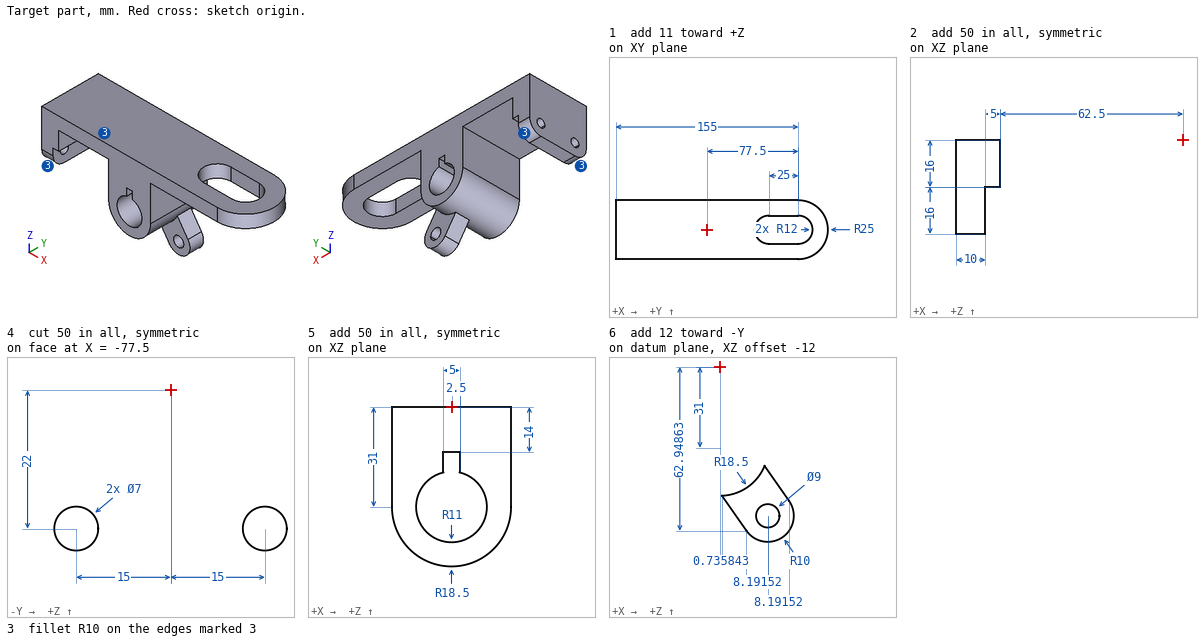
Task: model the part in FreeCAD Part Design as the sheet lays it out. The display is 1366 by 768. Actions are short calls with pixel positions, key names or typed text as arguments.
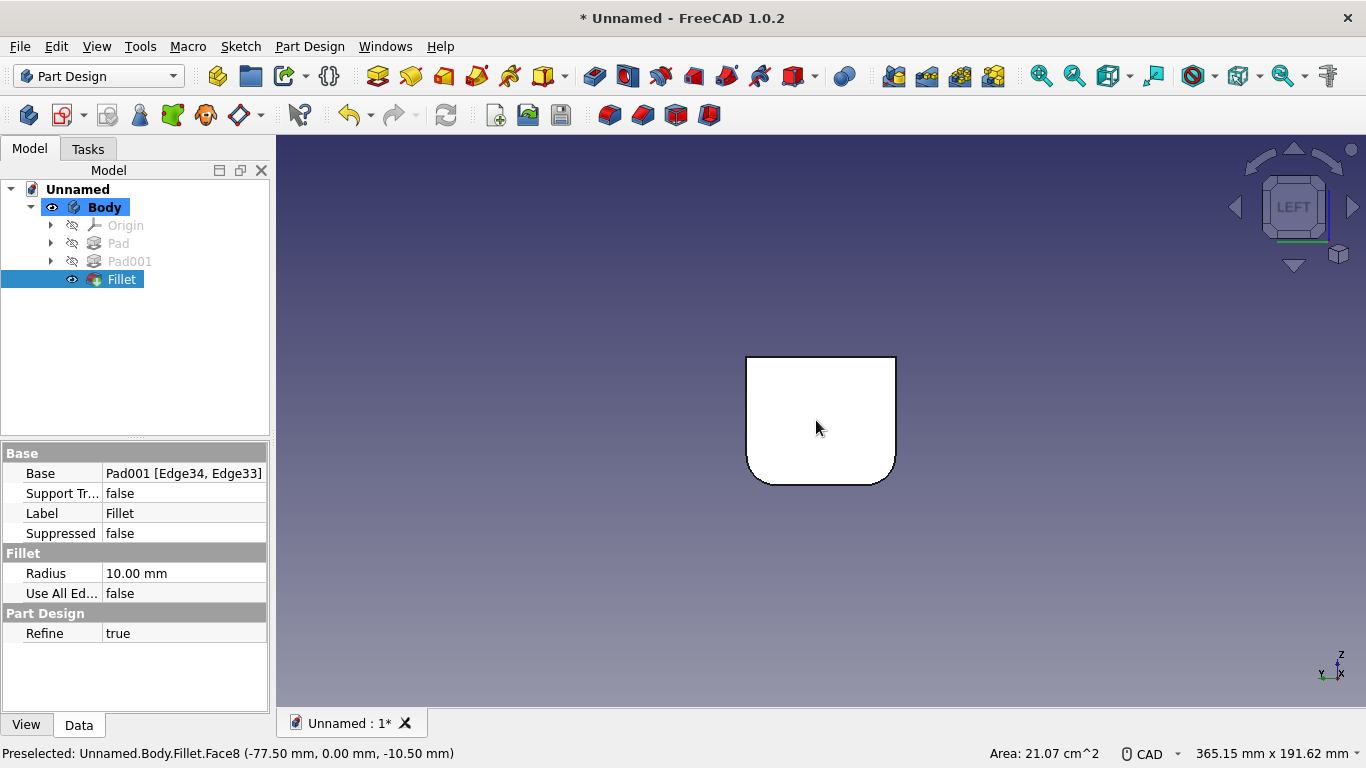
click(62, 116)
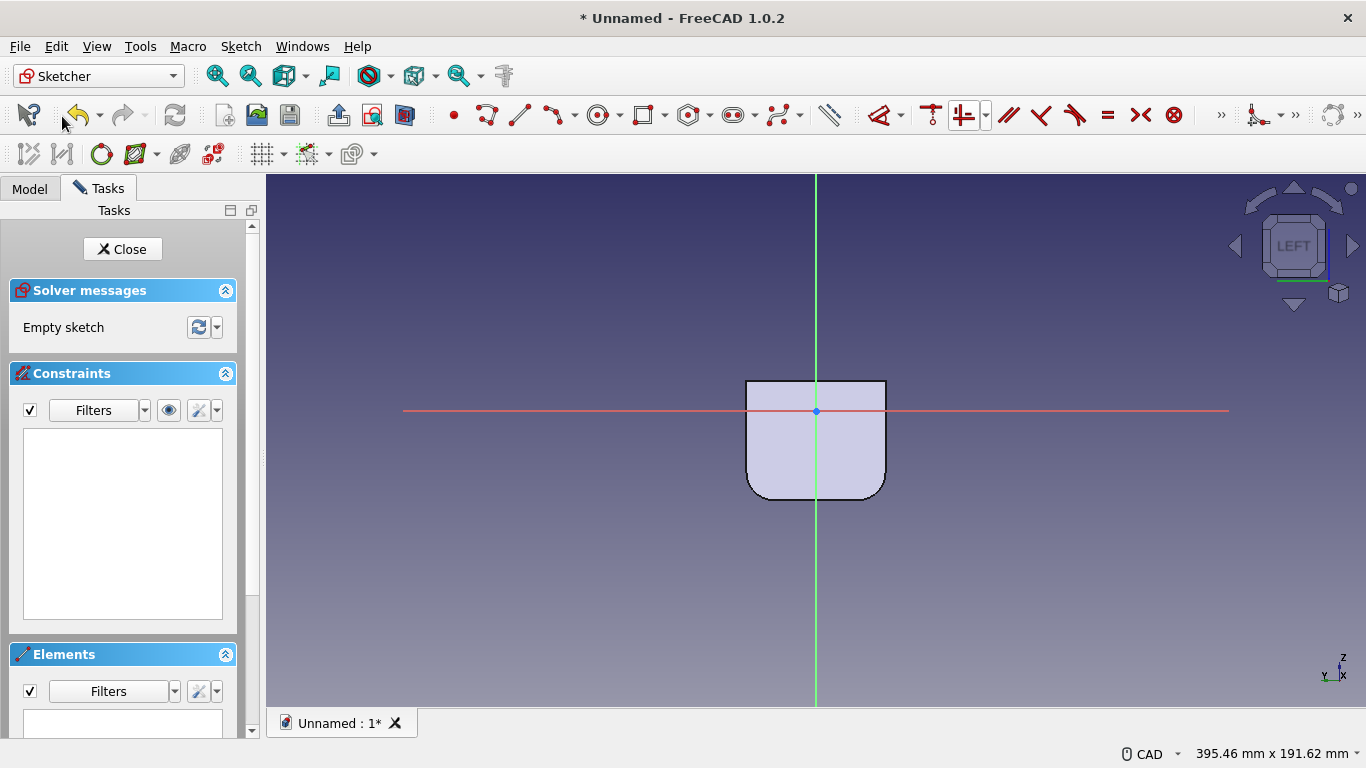
scroll(833, 448, up, 8)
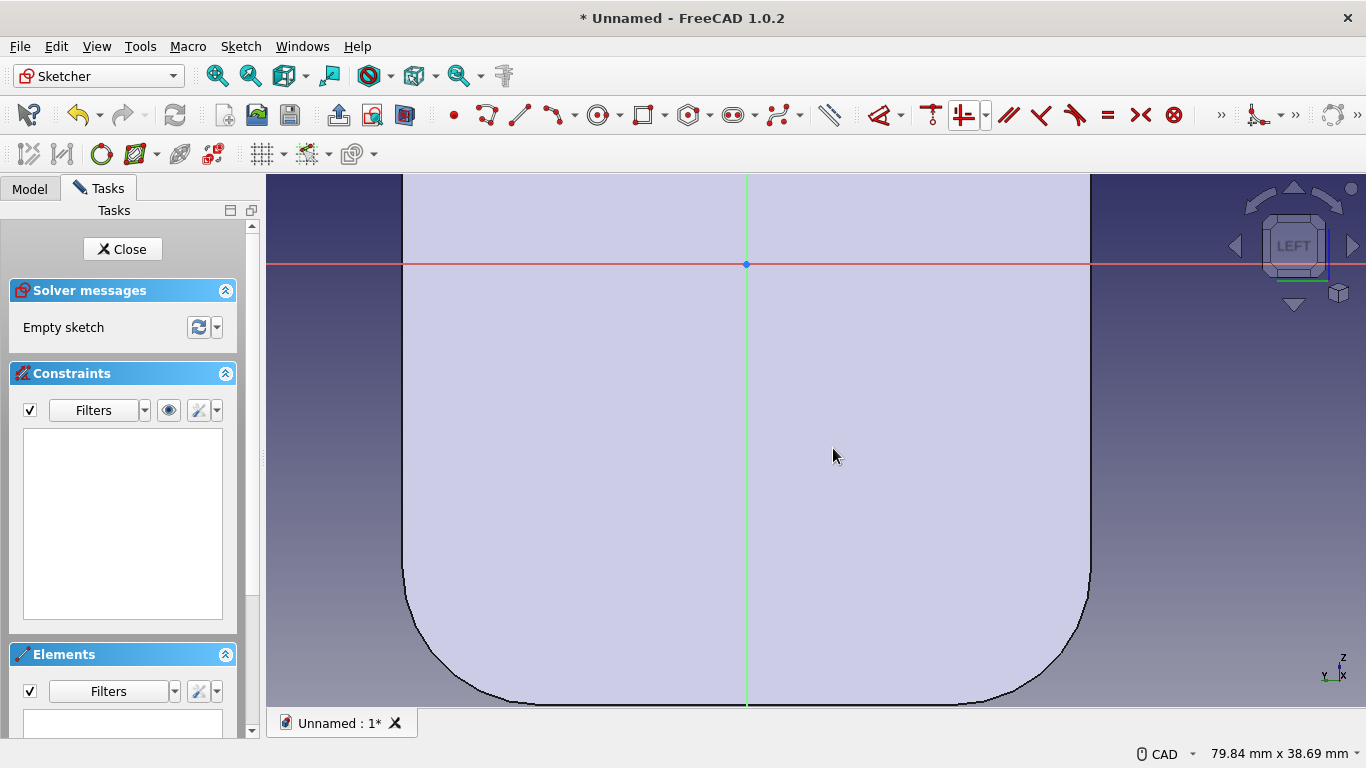
click(598, 116)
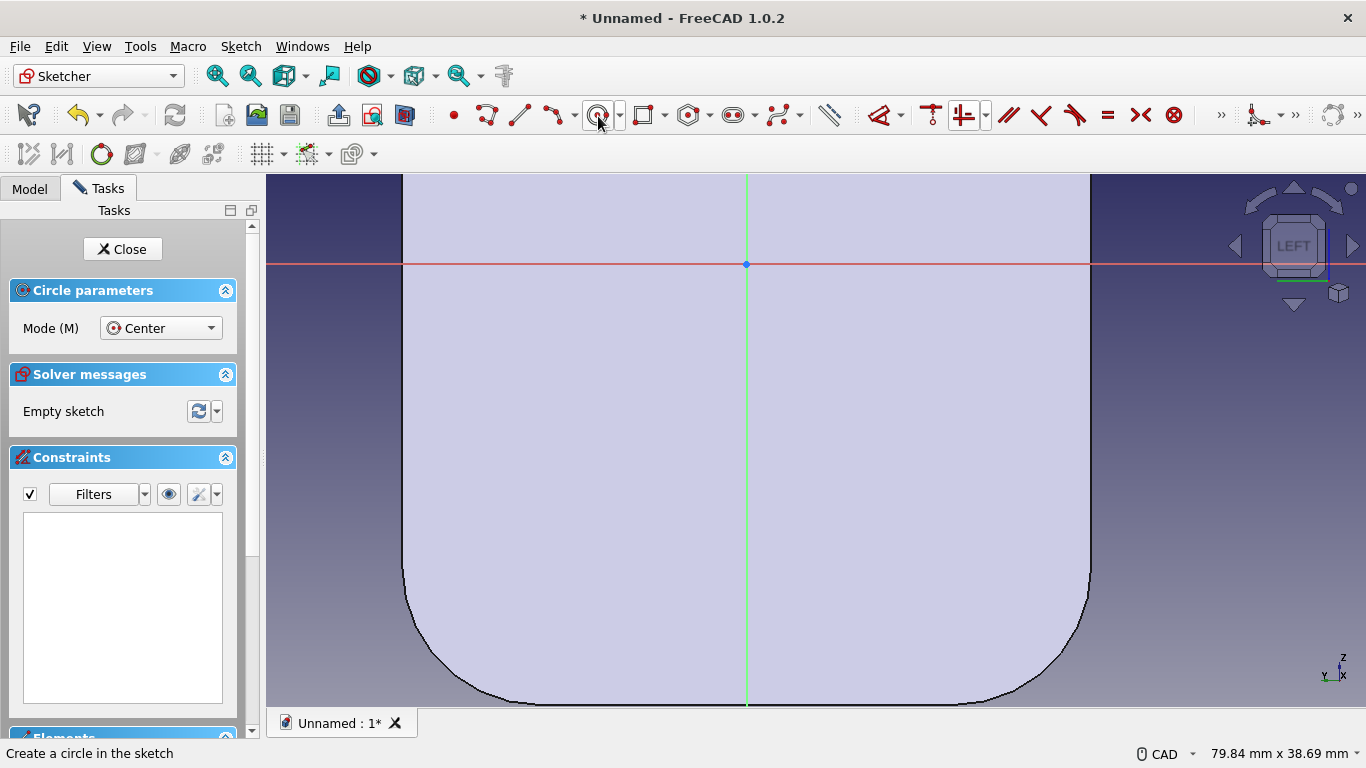
click(540, 567)
click(574, 533)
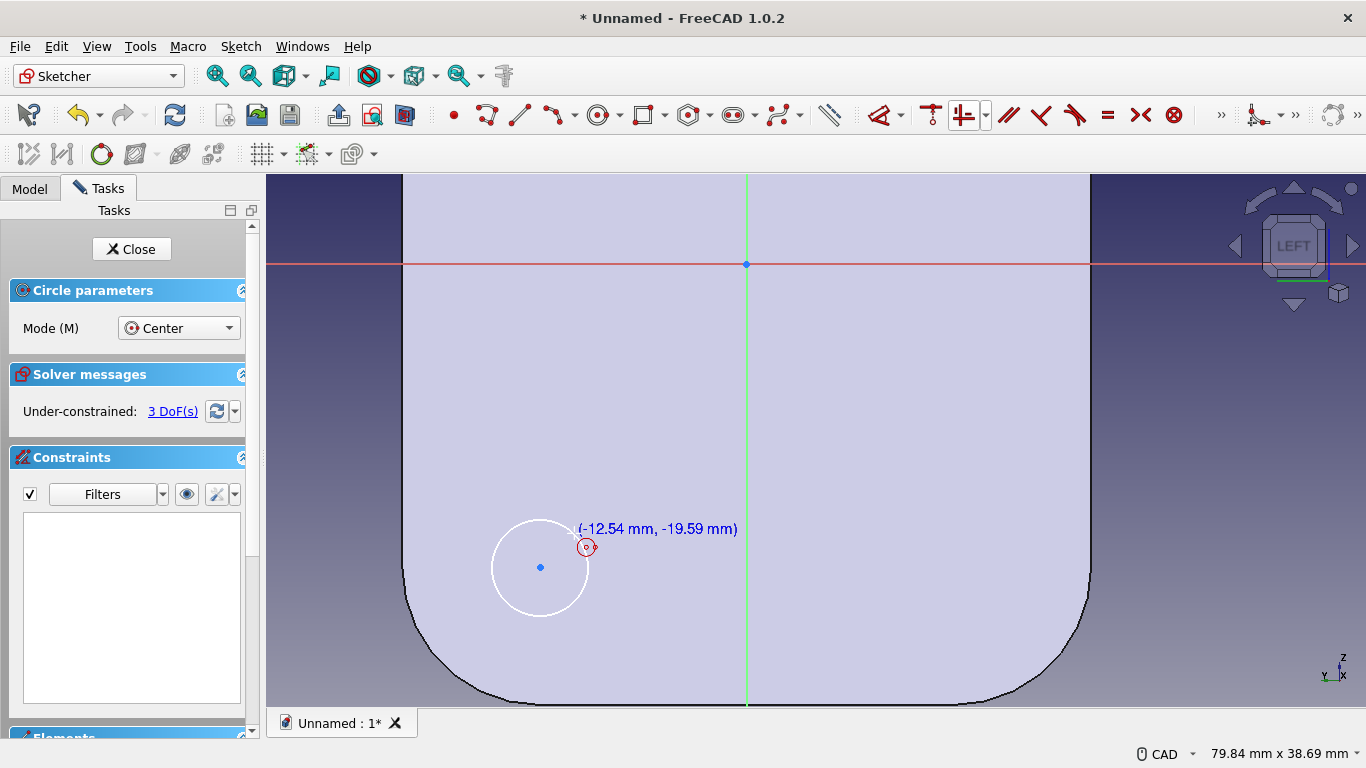
click(953, 567)
click(988, 533)
key(Escape)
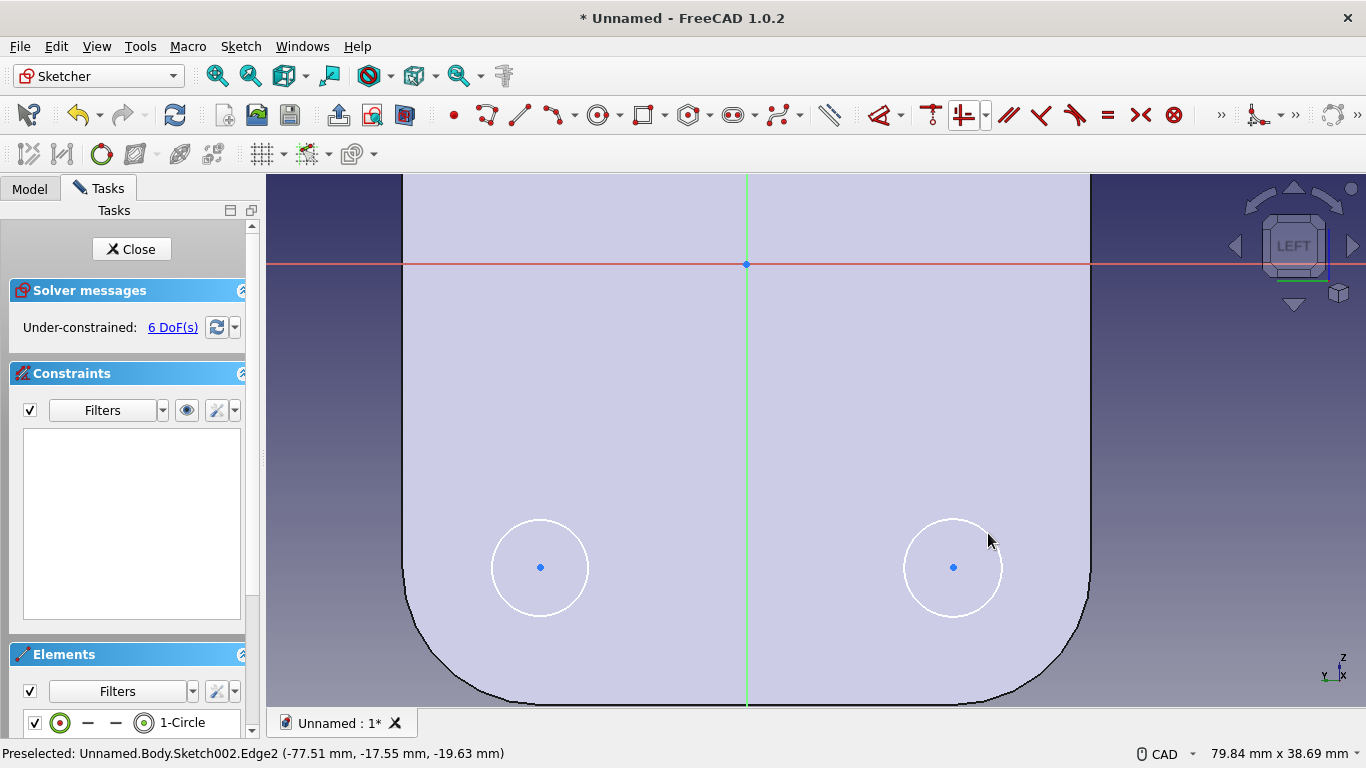
click(574, 534)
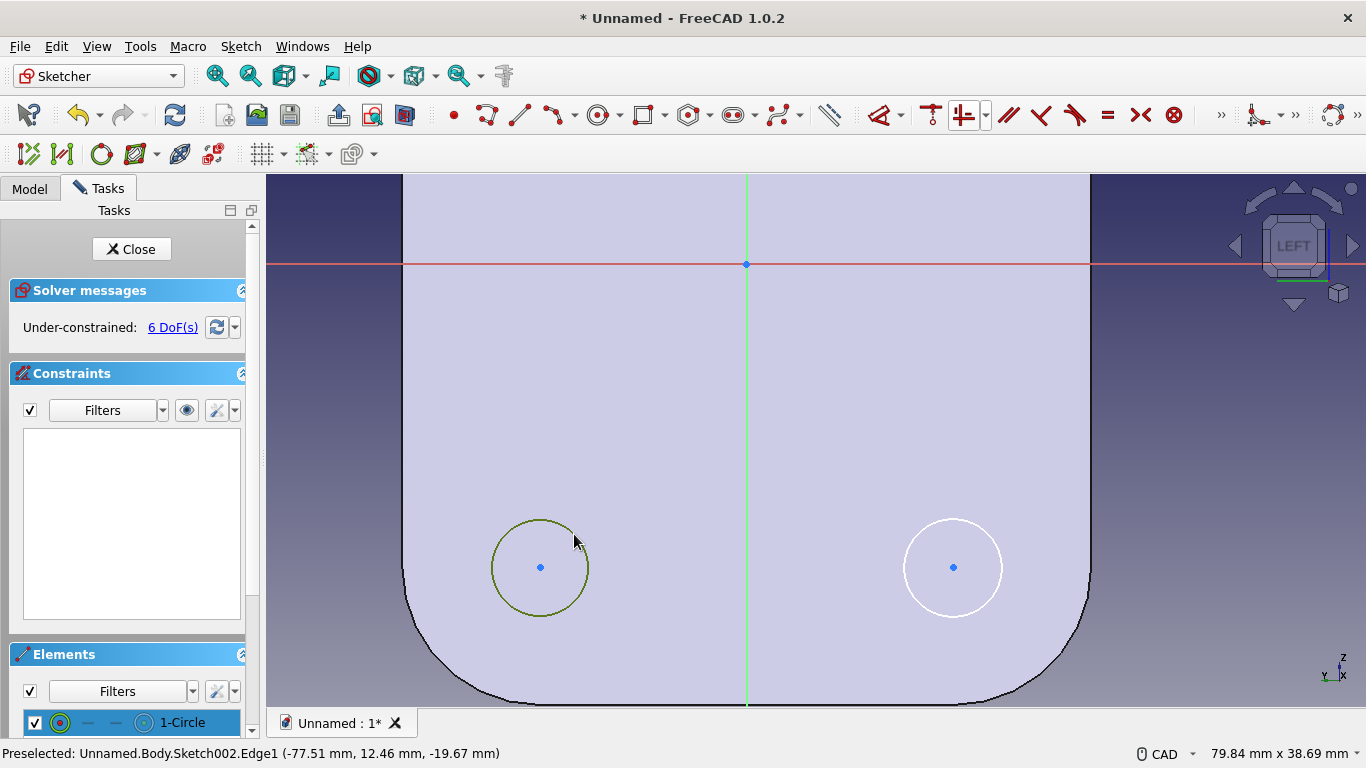
click(987, 533)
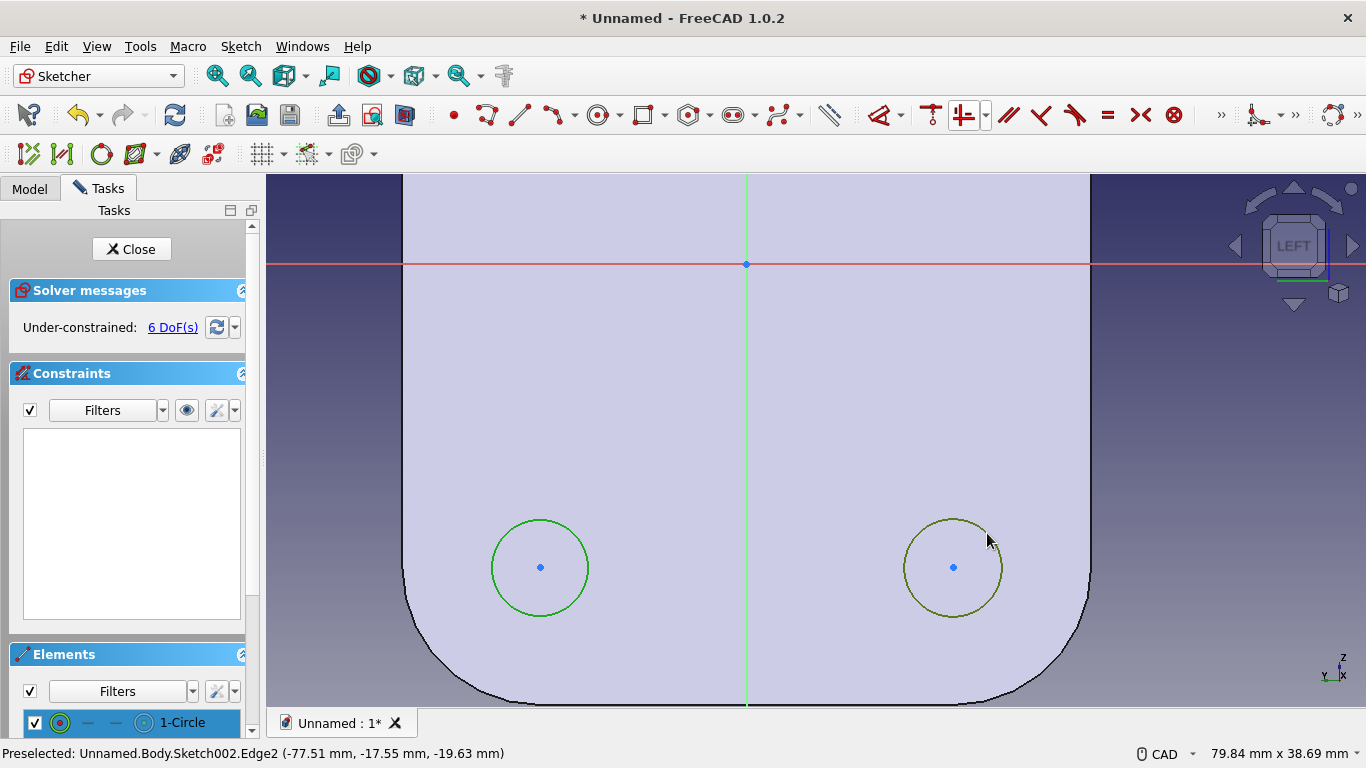
key(e)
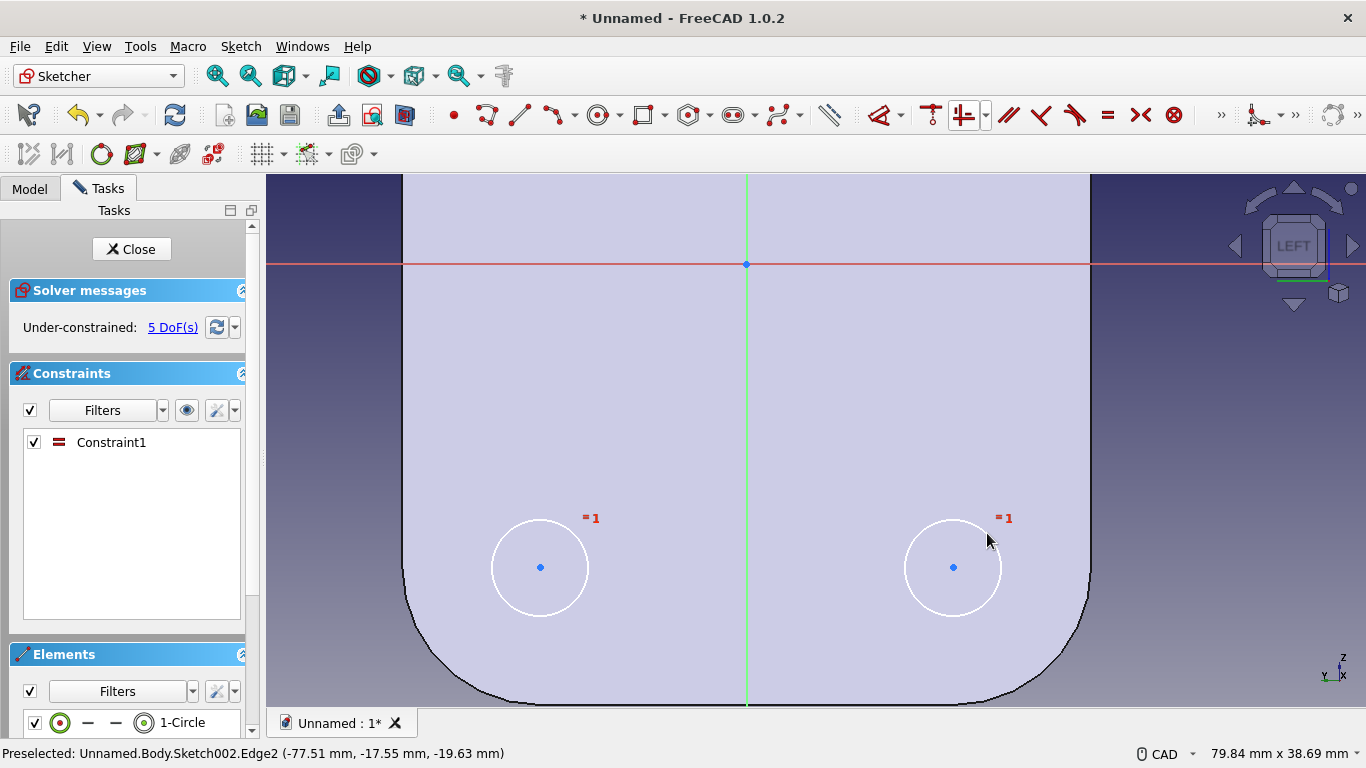
click(540, 568)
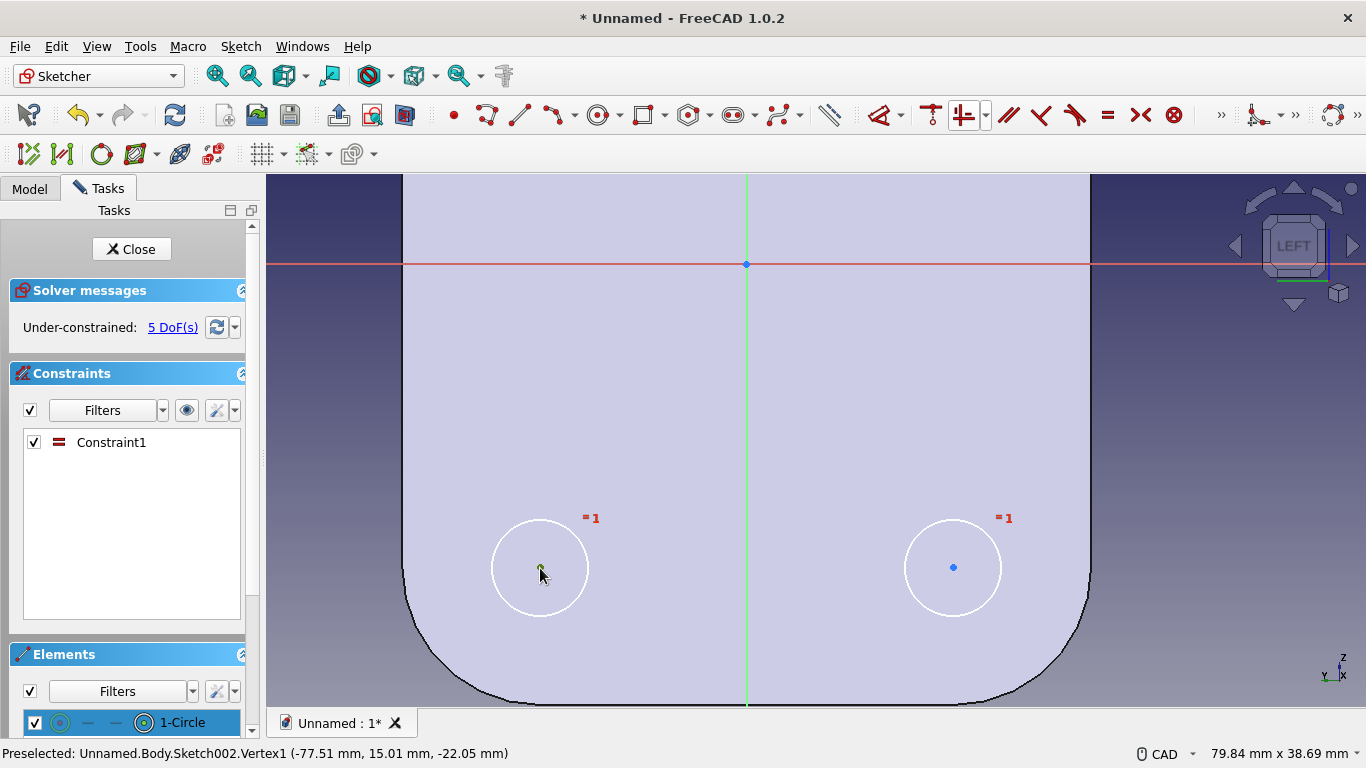
click(953, 568)